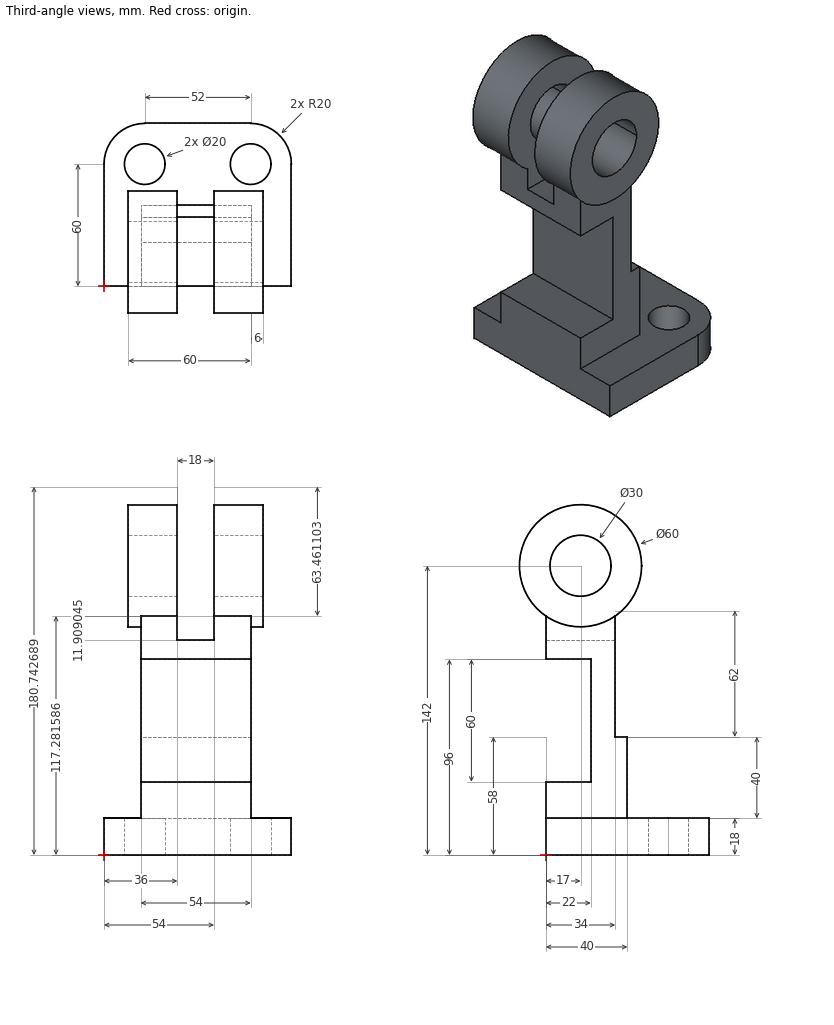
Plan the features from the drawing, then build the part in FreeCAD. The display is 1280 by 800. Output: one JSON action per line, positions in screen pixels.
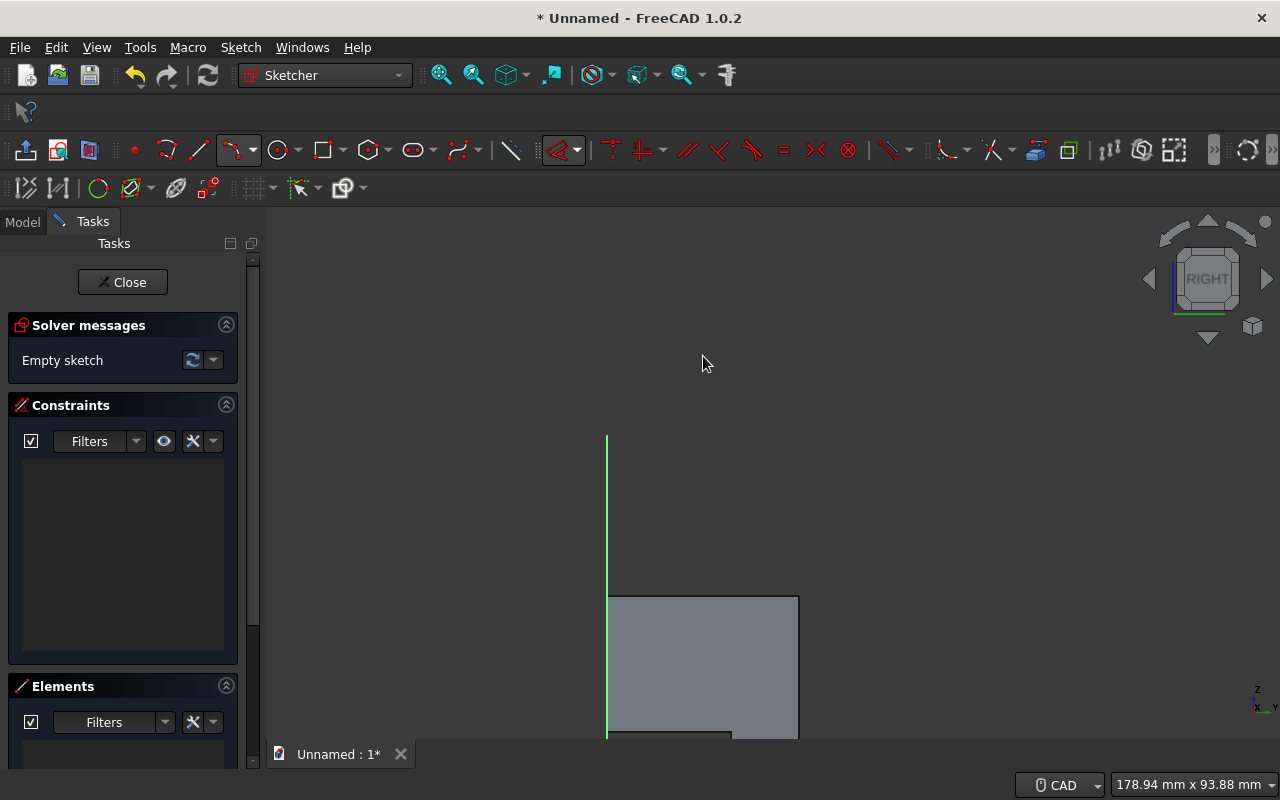
{"action": "left_click", "coordinate": [278, 150]}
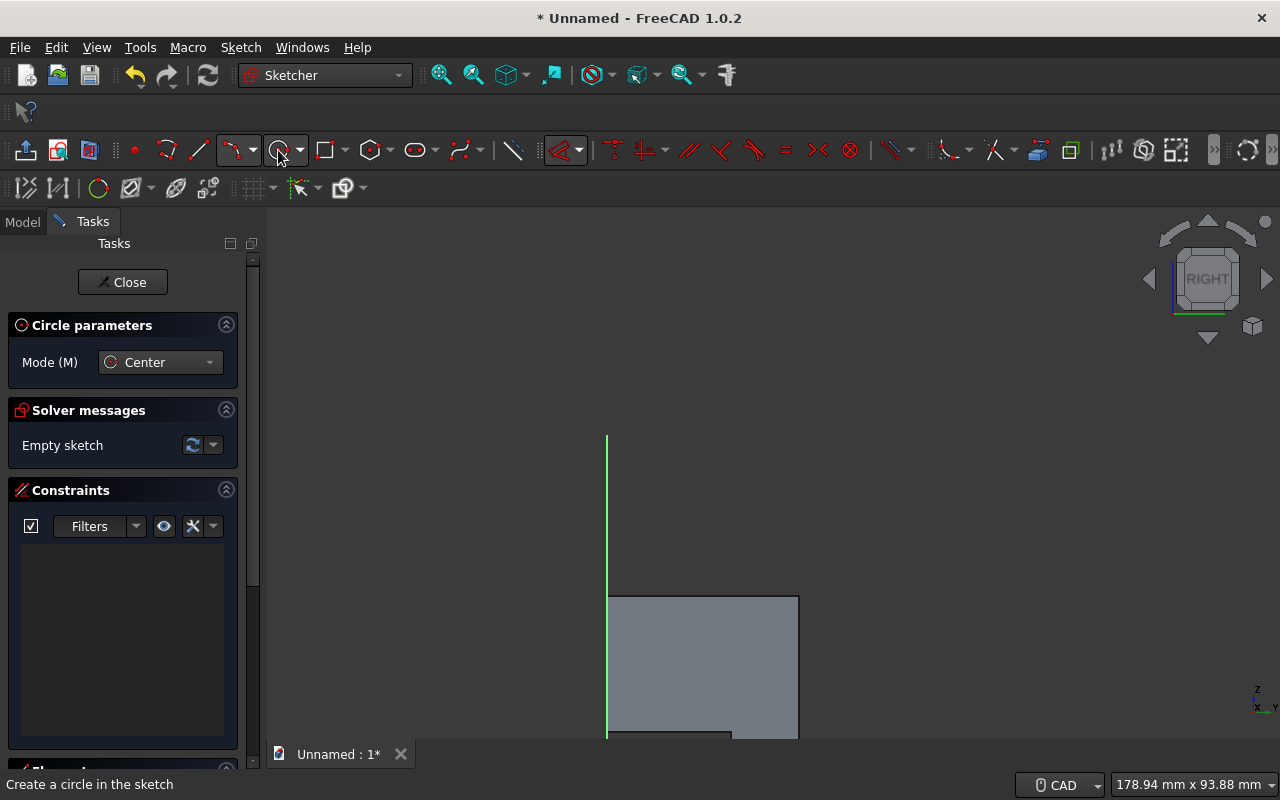
{"action": "left_click", "coordinate": [703, 471]}
{"action": "mouse_move", "coordinate": [823, 351]}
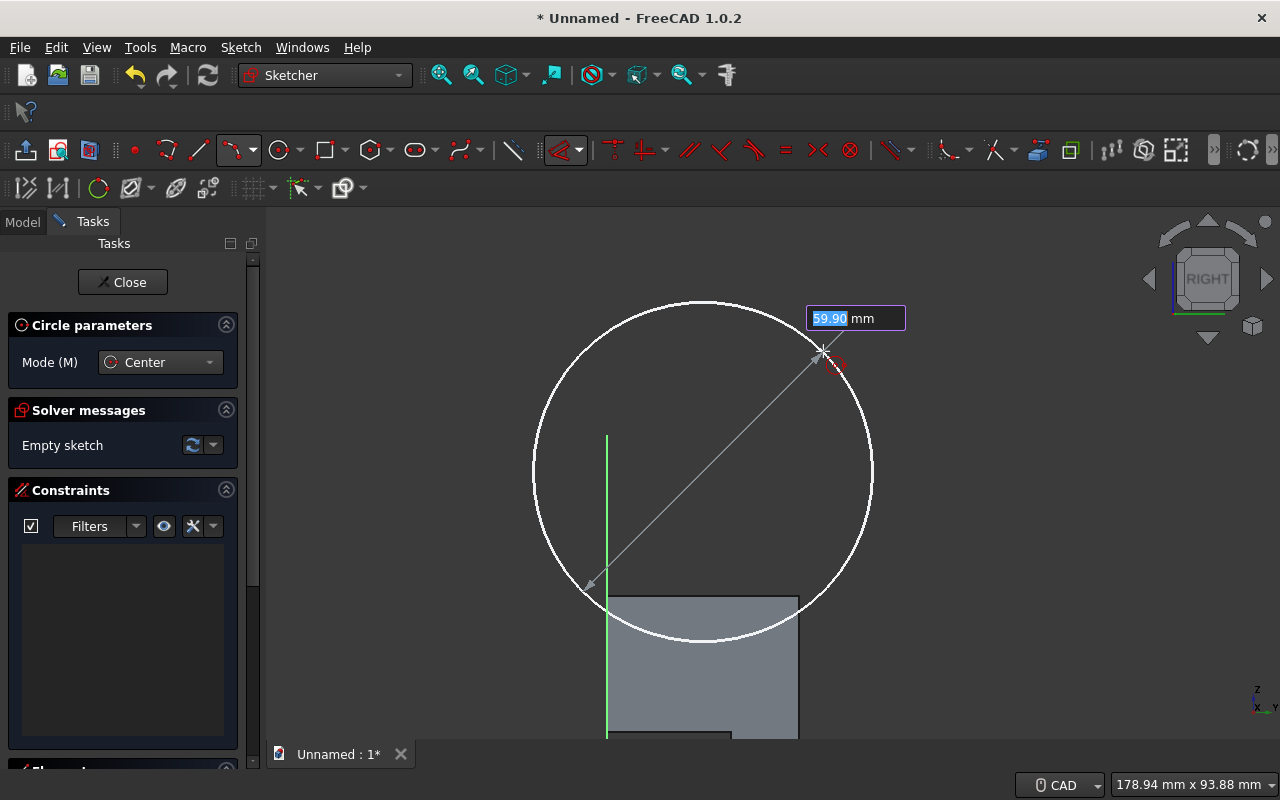
{"action": "type", "text": "60"}
{"action": "key", "text": "Return"}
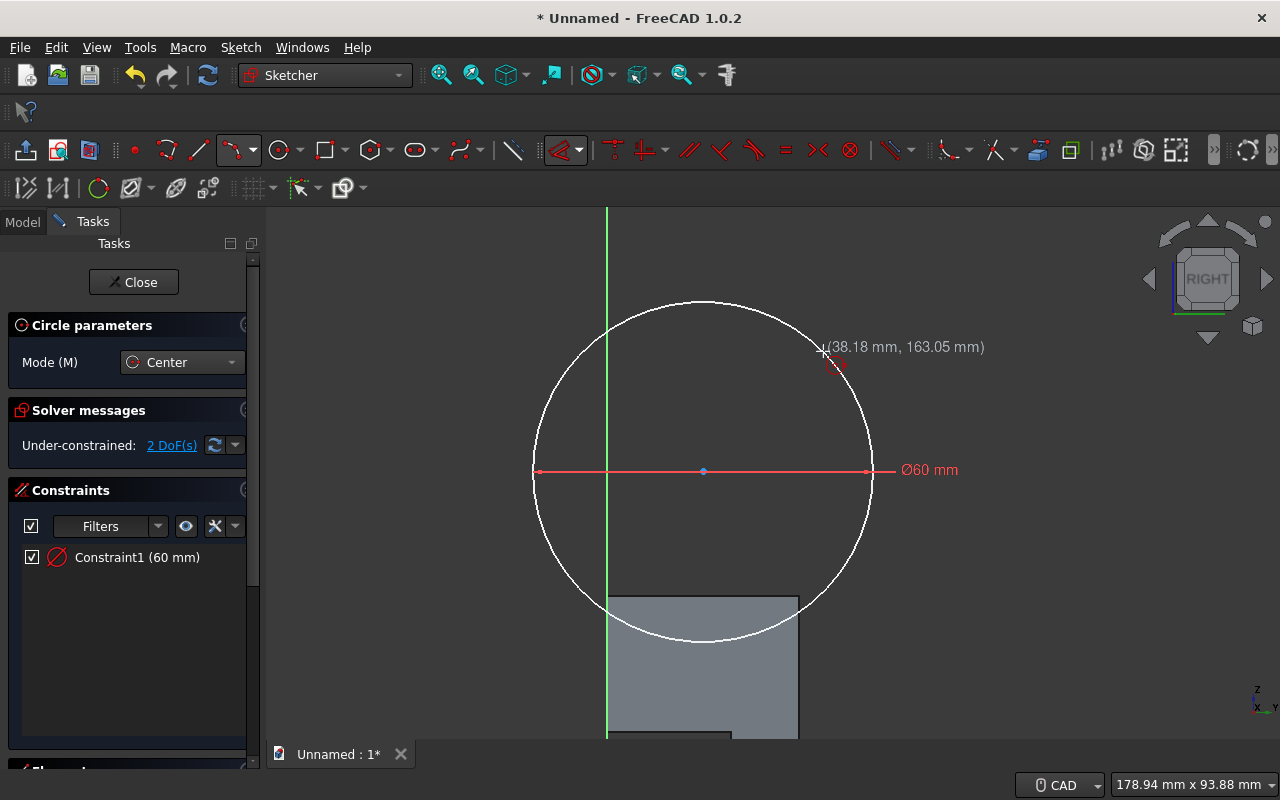
{"action": "left_click", "coordinate": [703, 472]}
{"action": "mouse_move", "coordinate": [763, 411]}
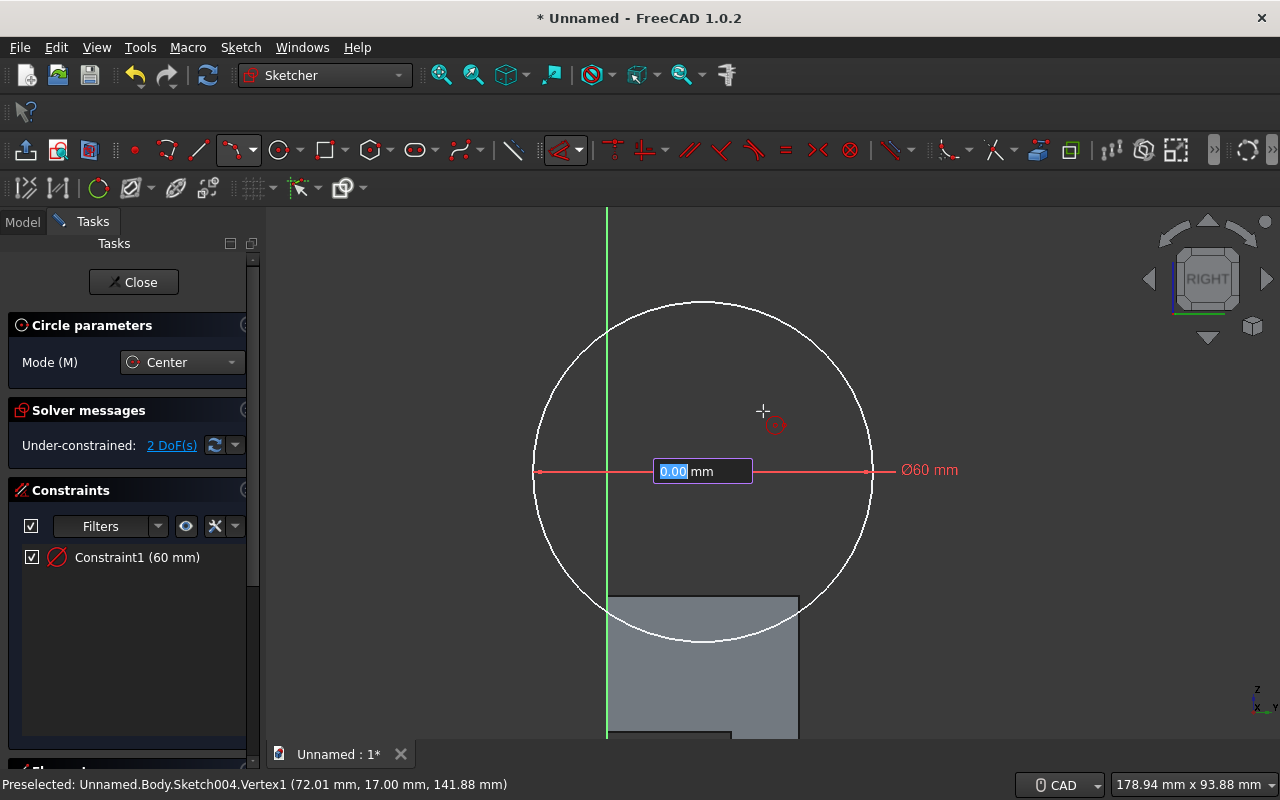
{"action": "type", "text": "30"}
{"action": "key", "text": "Return"}
{"action": "key", "text": "Escape"}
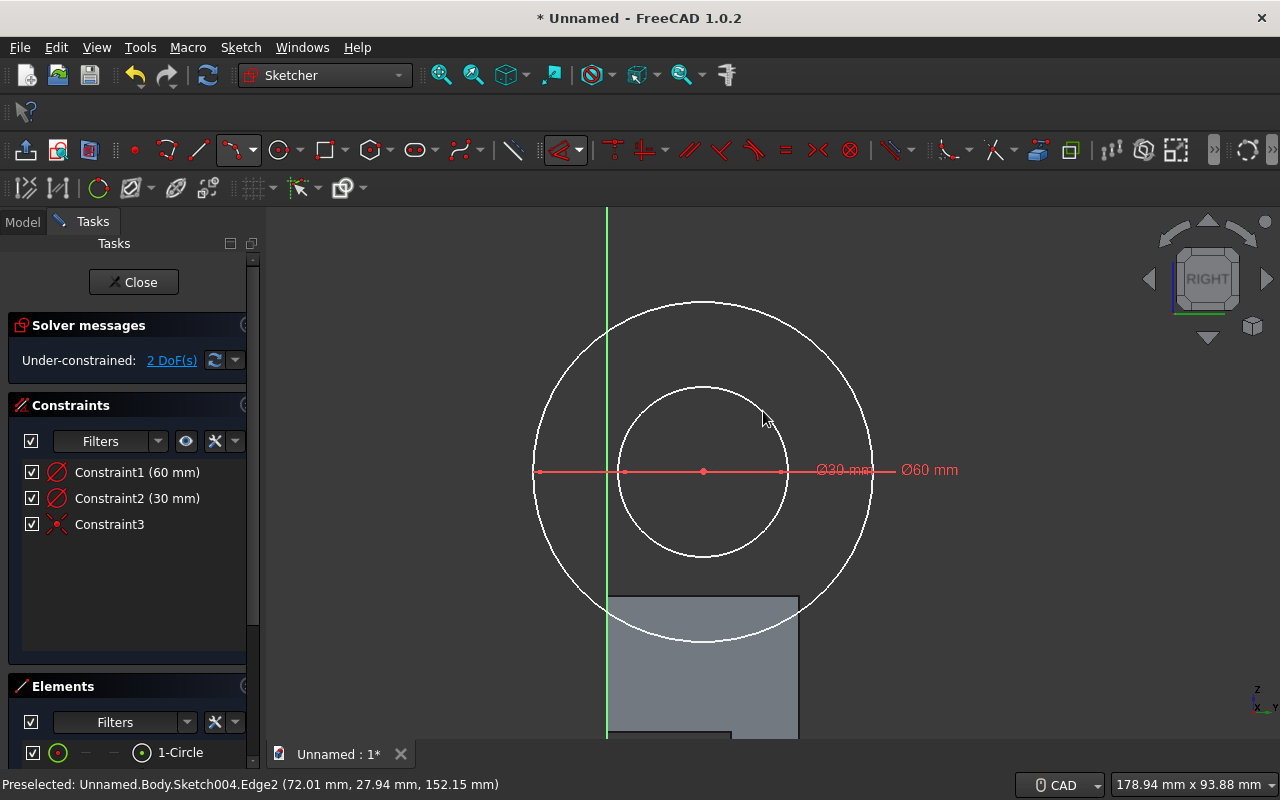
{"action": "left_click", "coordinate": [703, 472]}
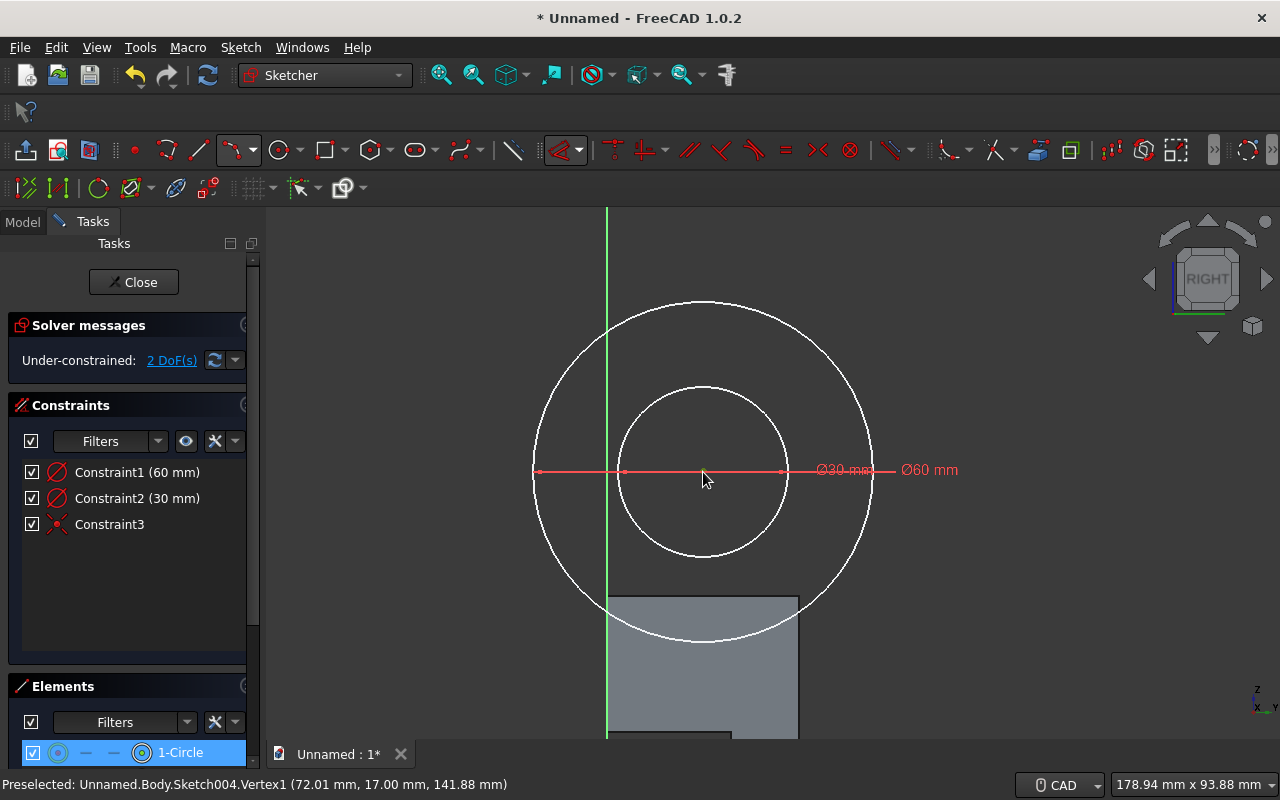
{"action": "left_click", "coordinate": [582, 150]}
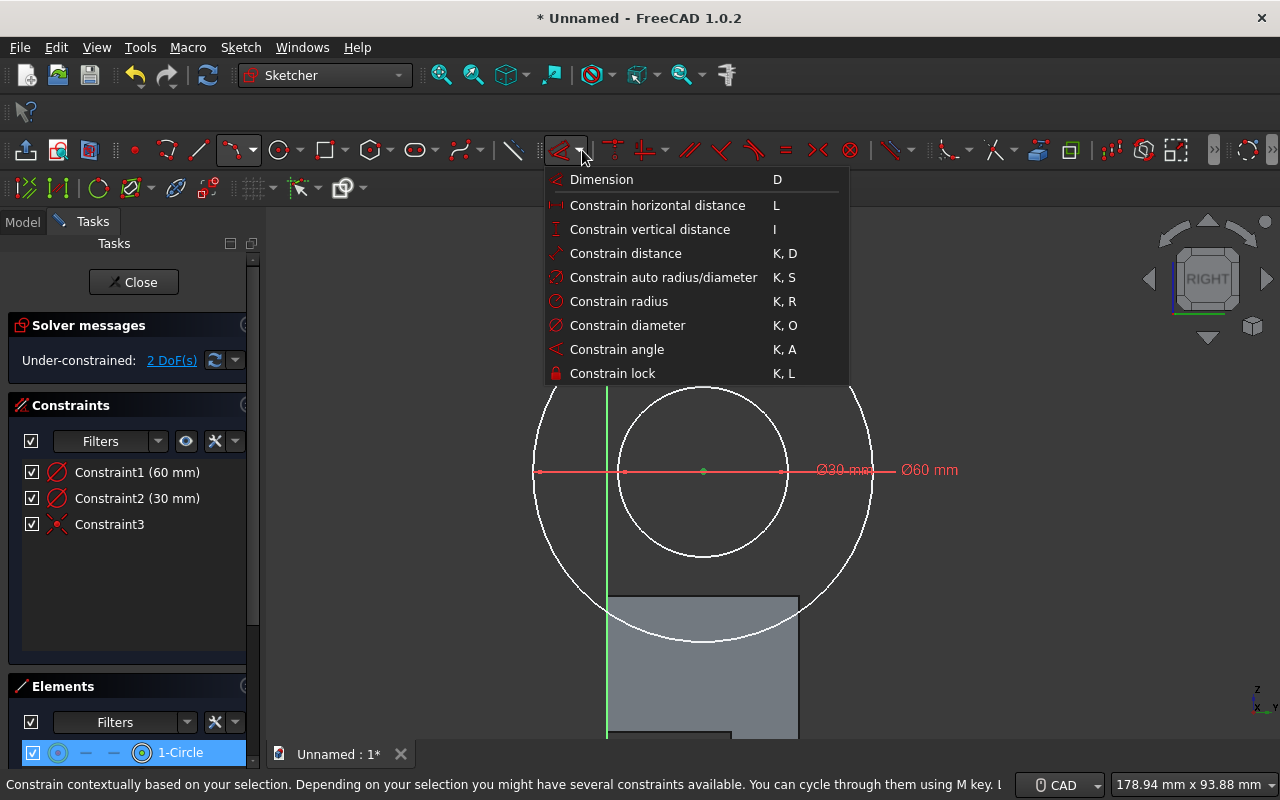
{"action": "left_click", "coordinate": [697, 205]}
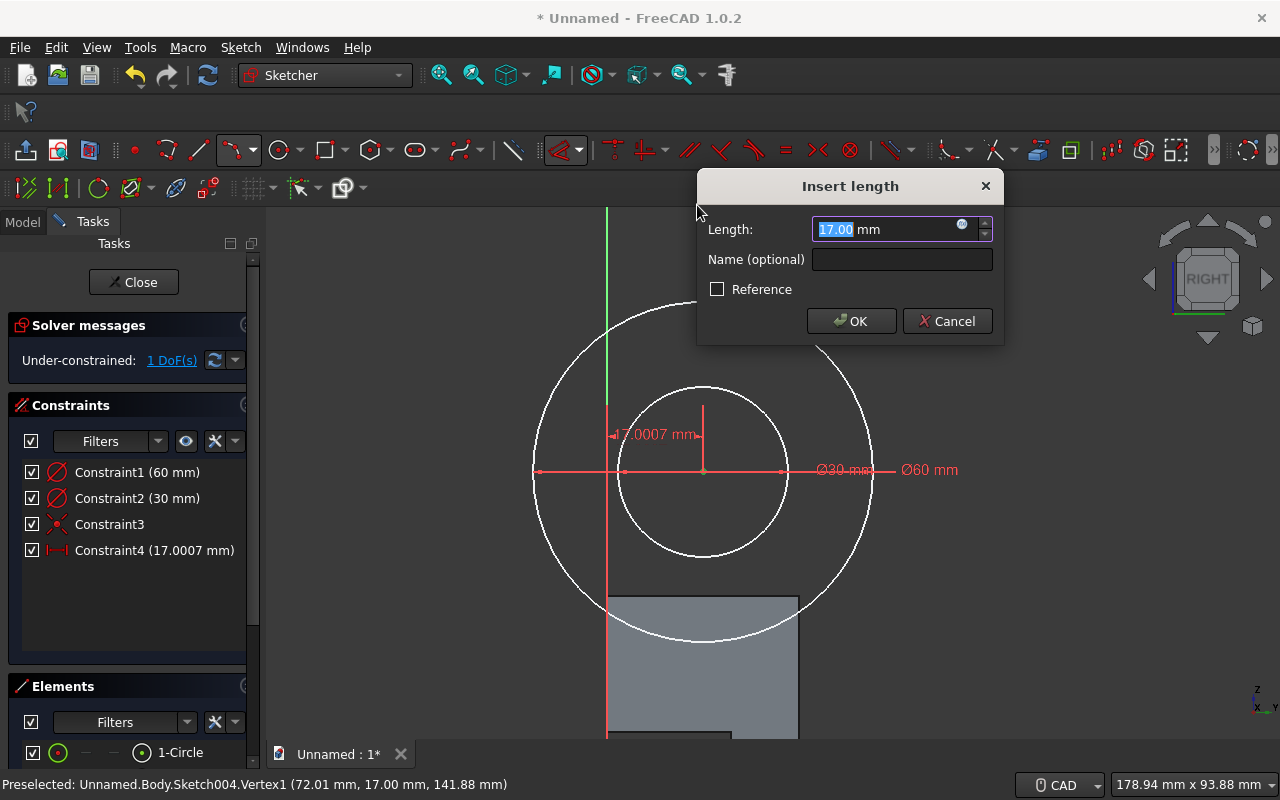
{"action": "type", "text": "17"}
{"action": "key", "text": "Return"}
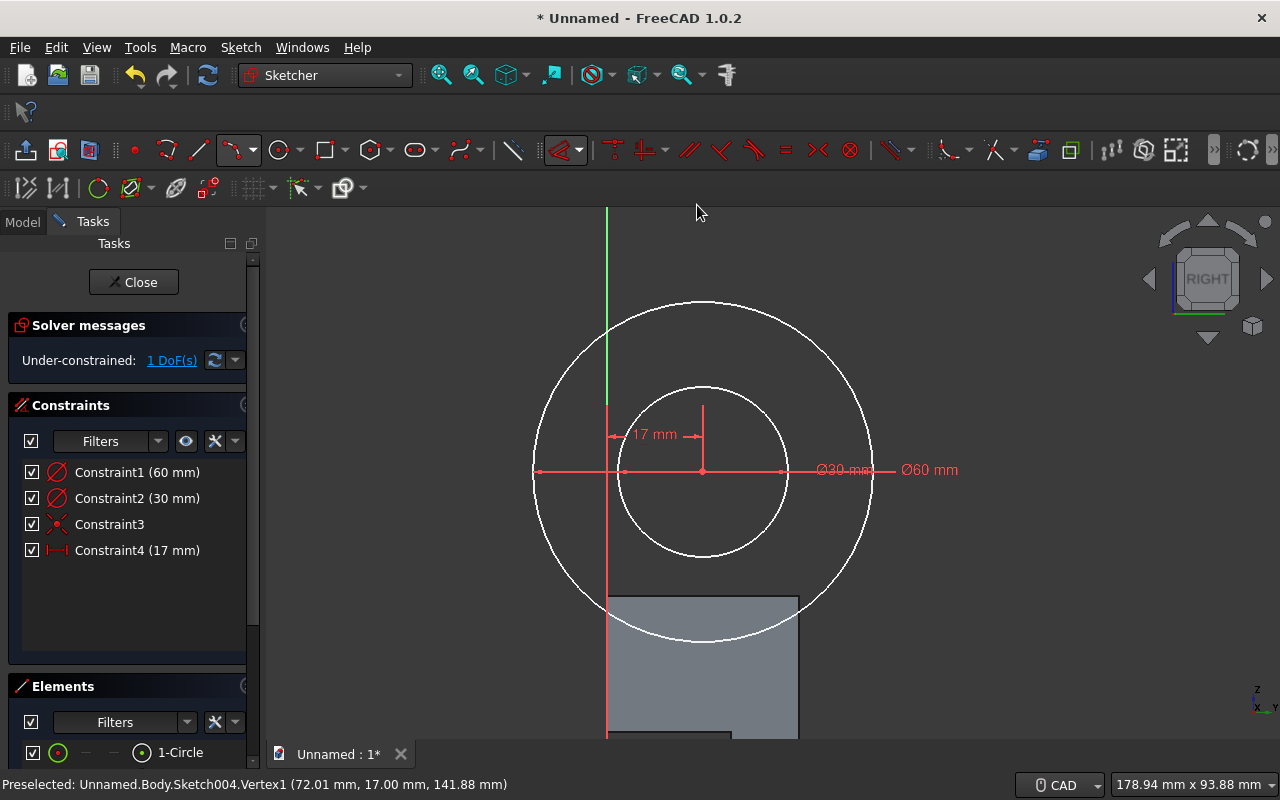
{"action": "left_click", "coordinate": [703, 472]}